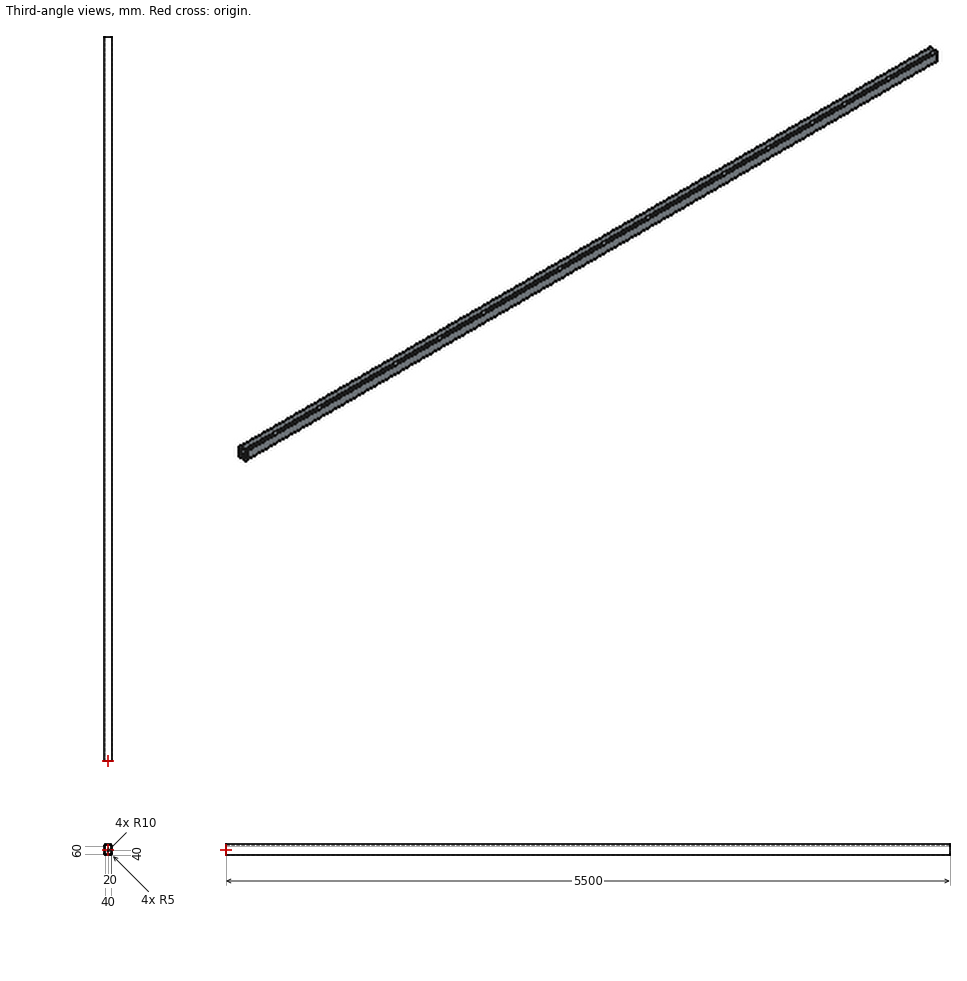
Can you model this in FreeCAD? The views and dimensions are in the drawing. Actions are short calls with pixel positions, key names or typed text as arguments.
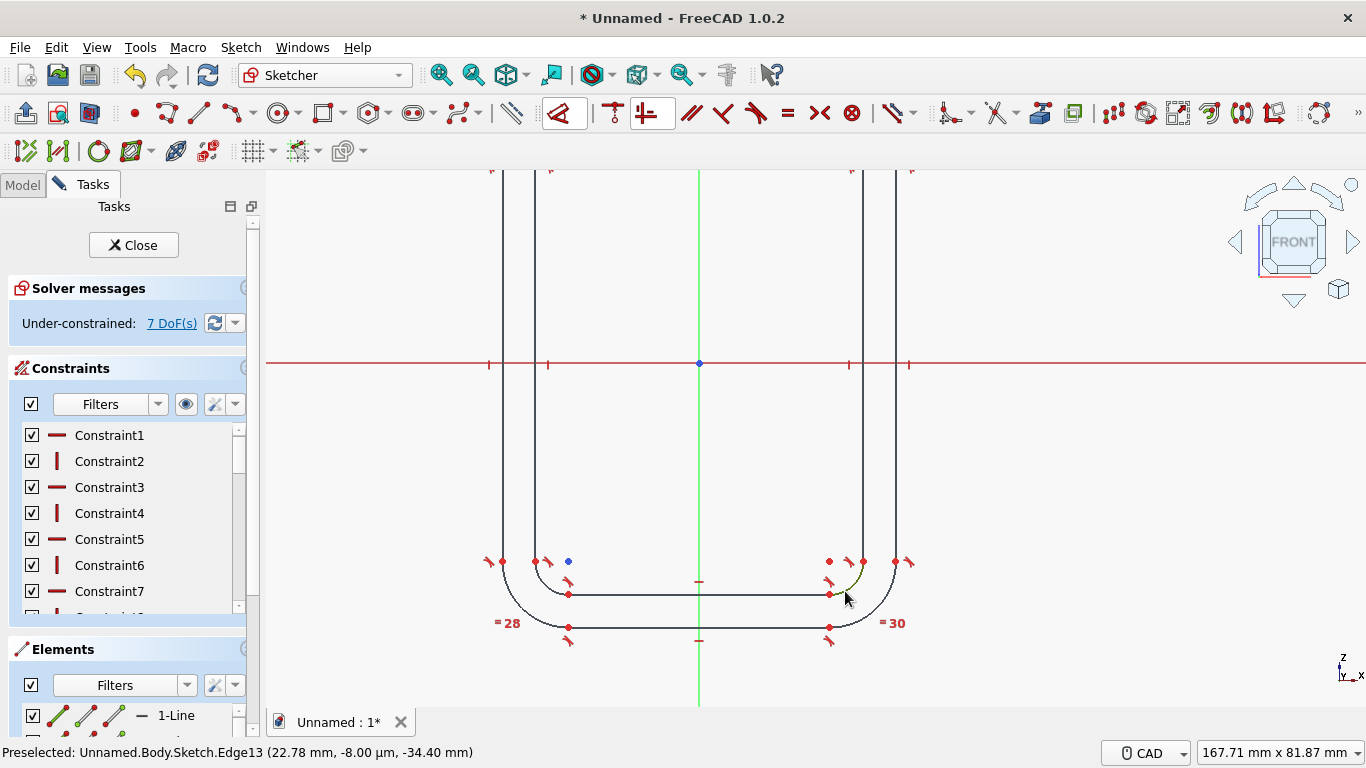
click(539, 577)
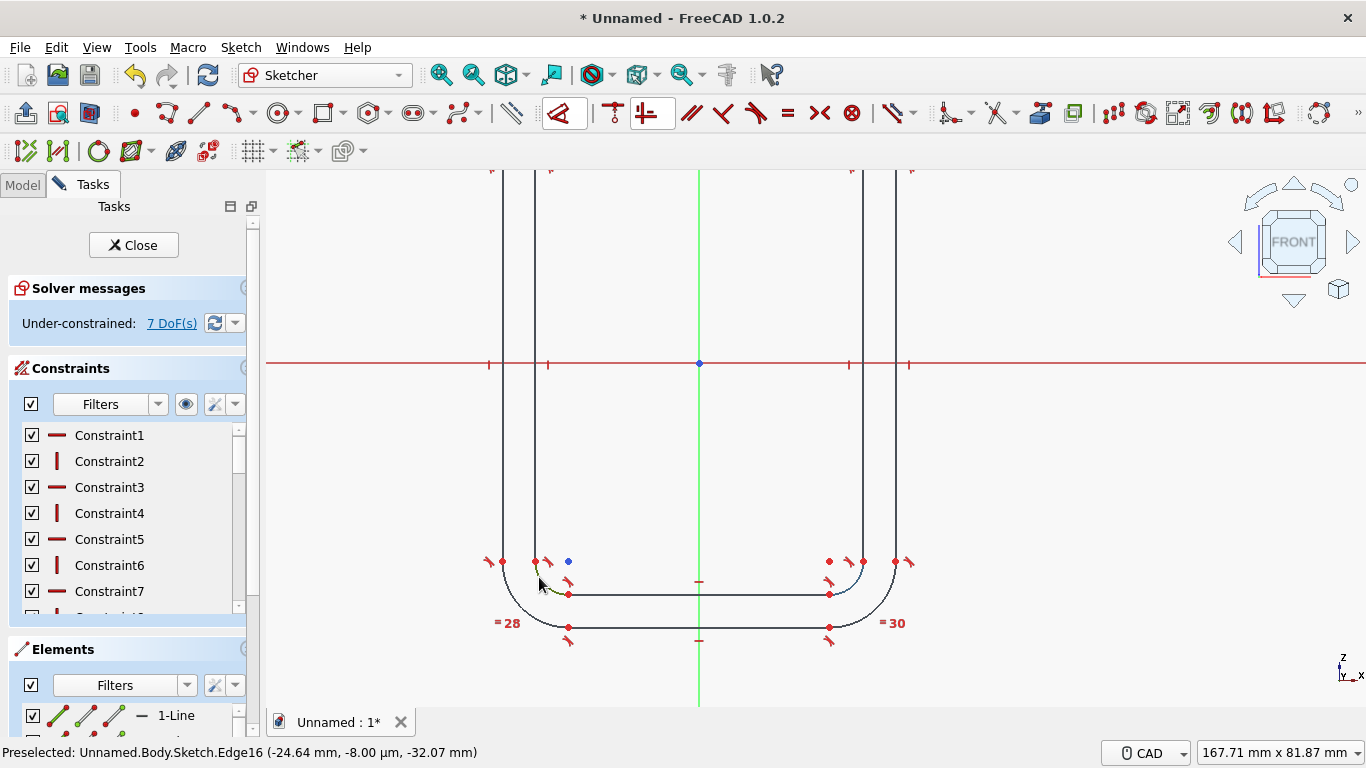
click(788, 114)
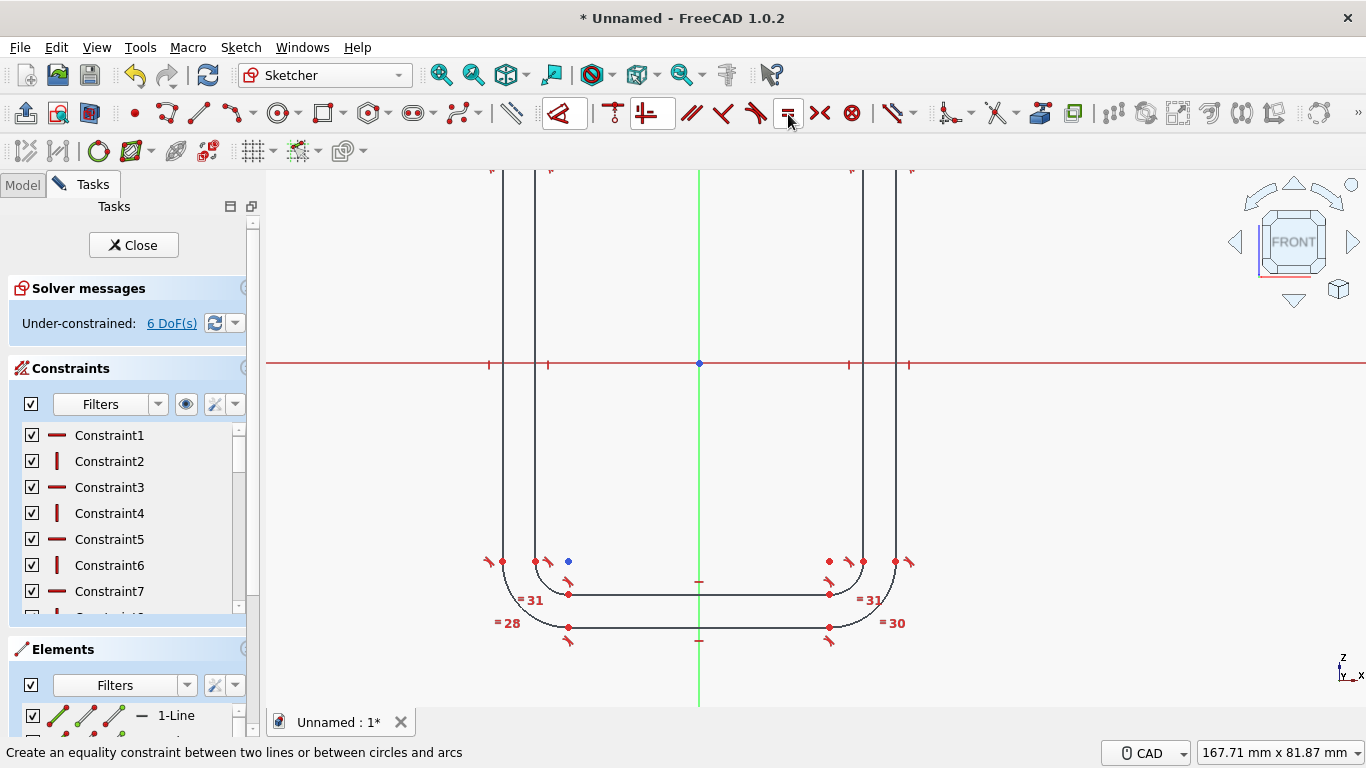
click(558, 114)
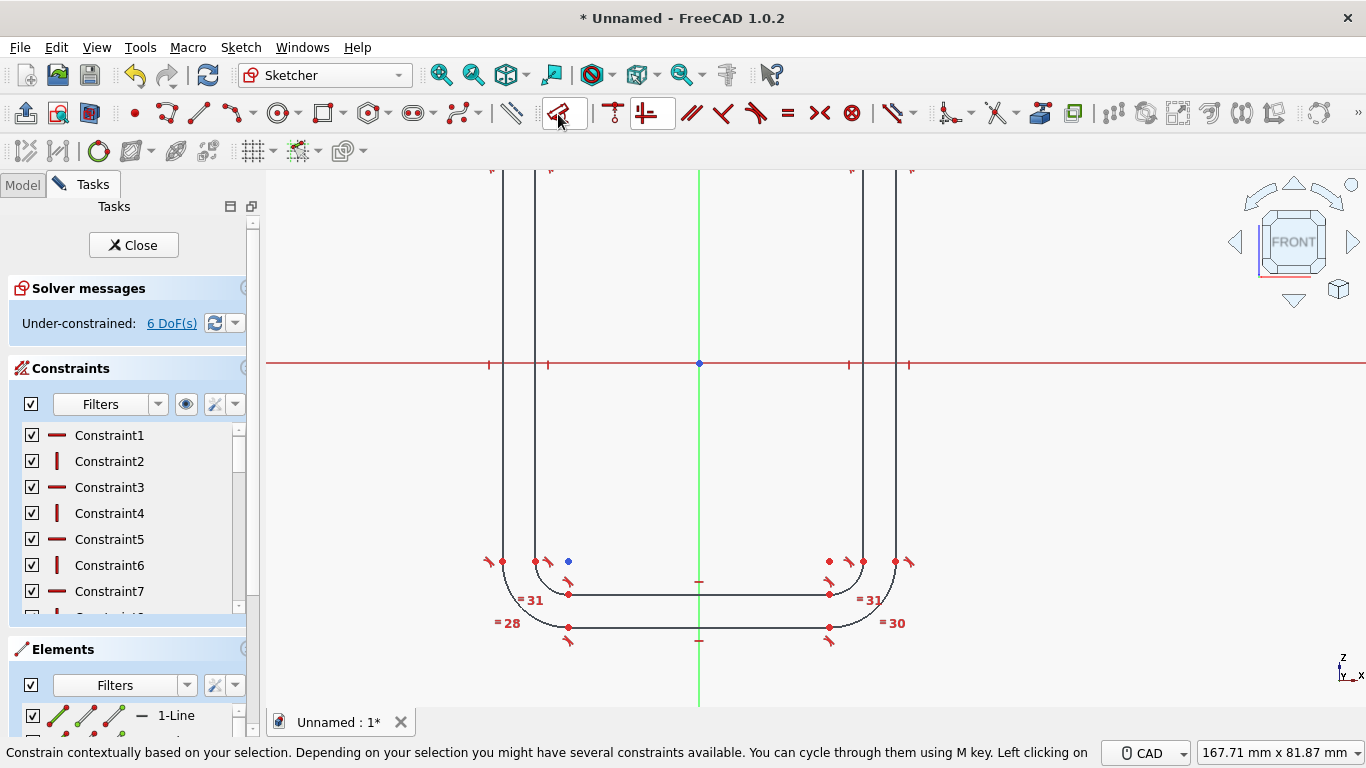
click(510, 592)
click(482, 607)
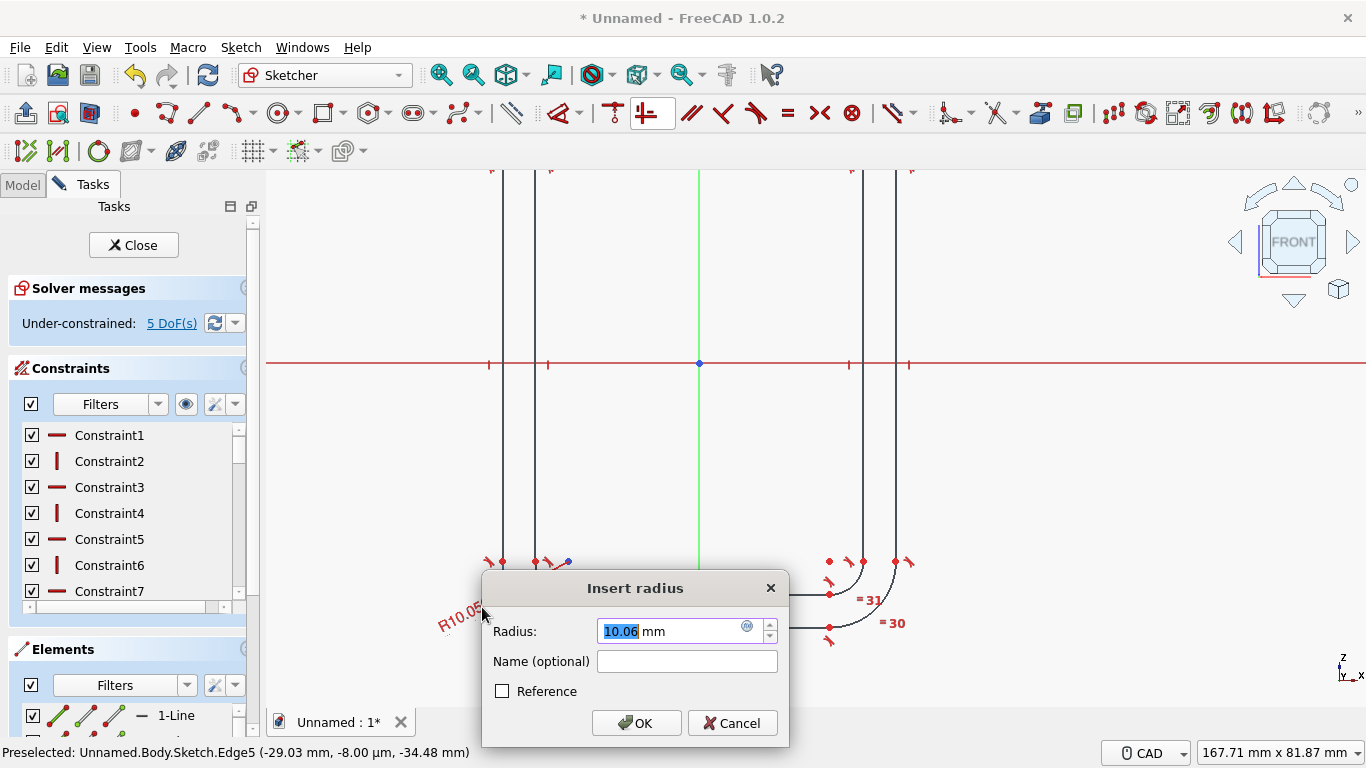
text(10)
key(Return)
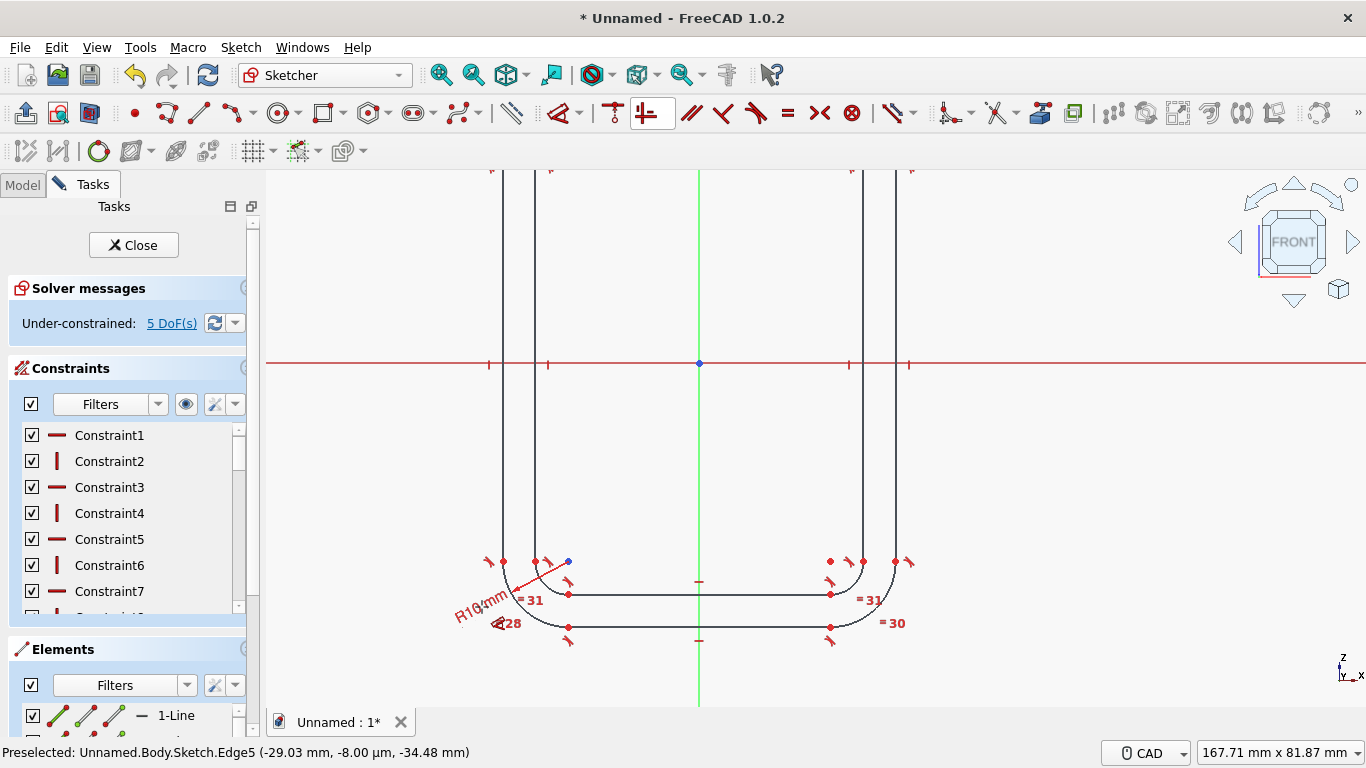
click(845, 591)
click(801, 504)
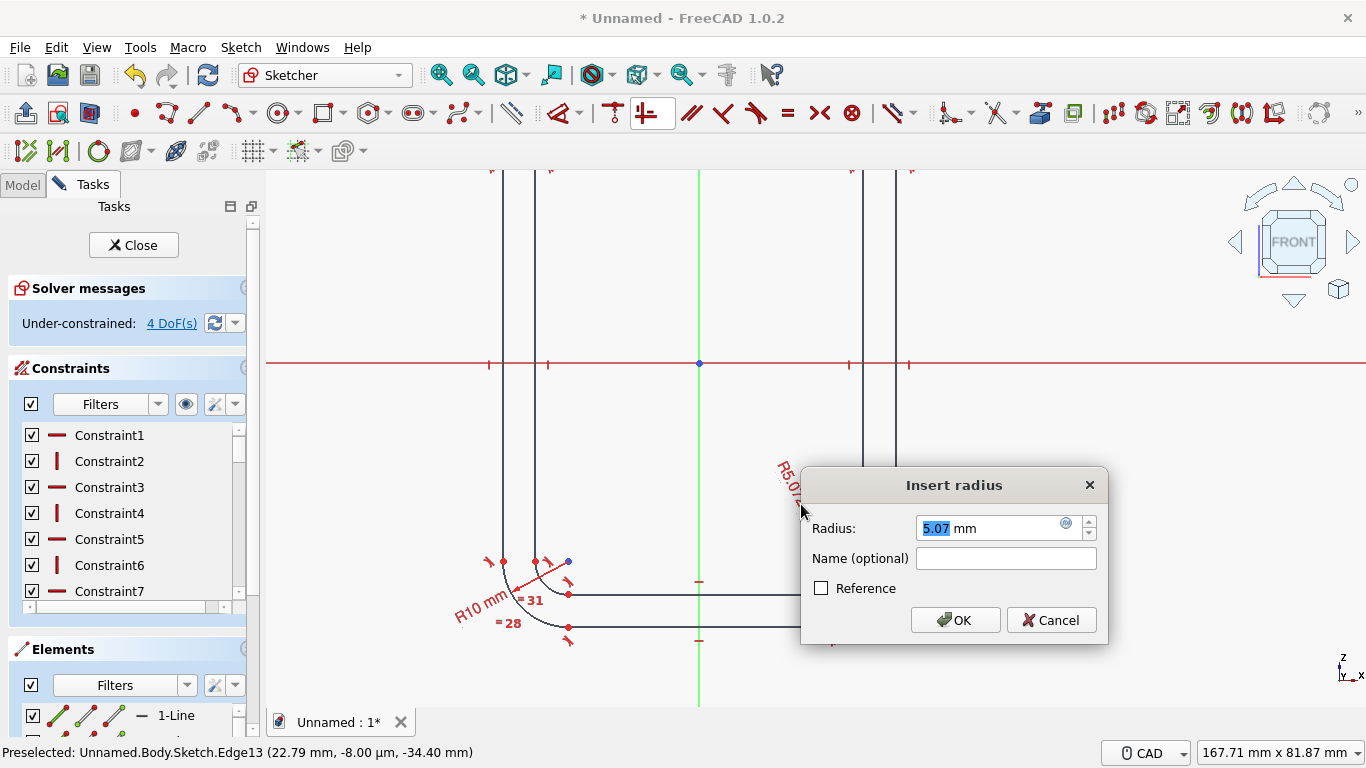
text(5)
key(Return)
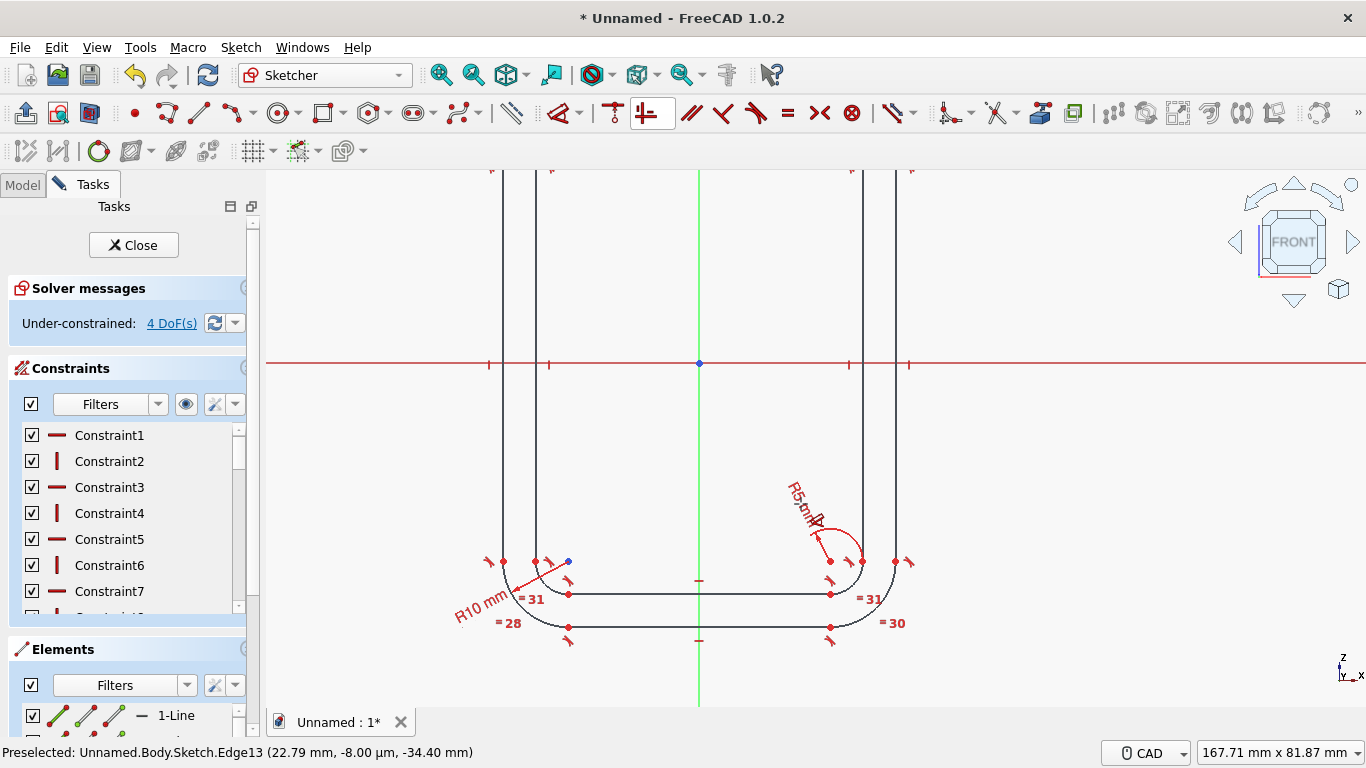
click(752, 627)
click(639, 661)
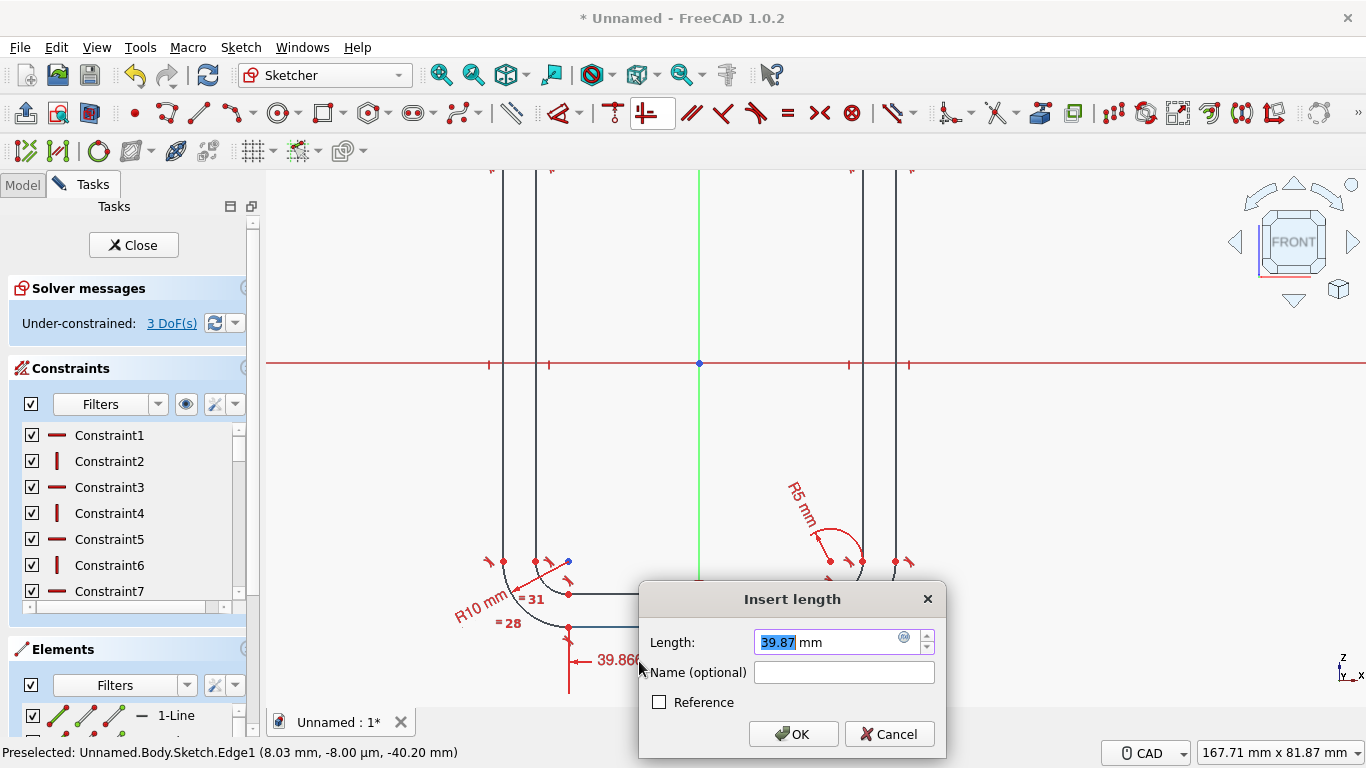
text(40)
key(Return)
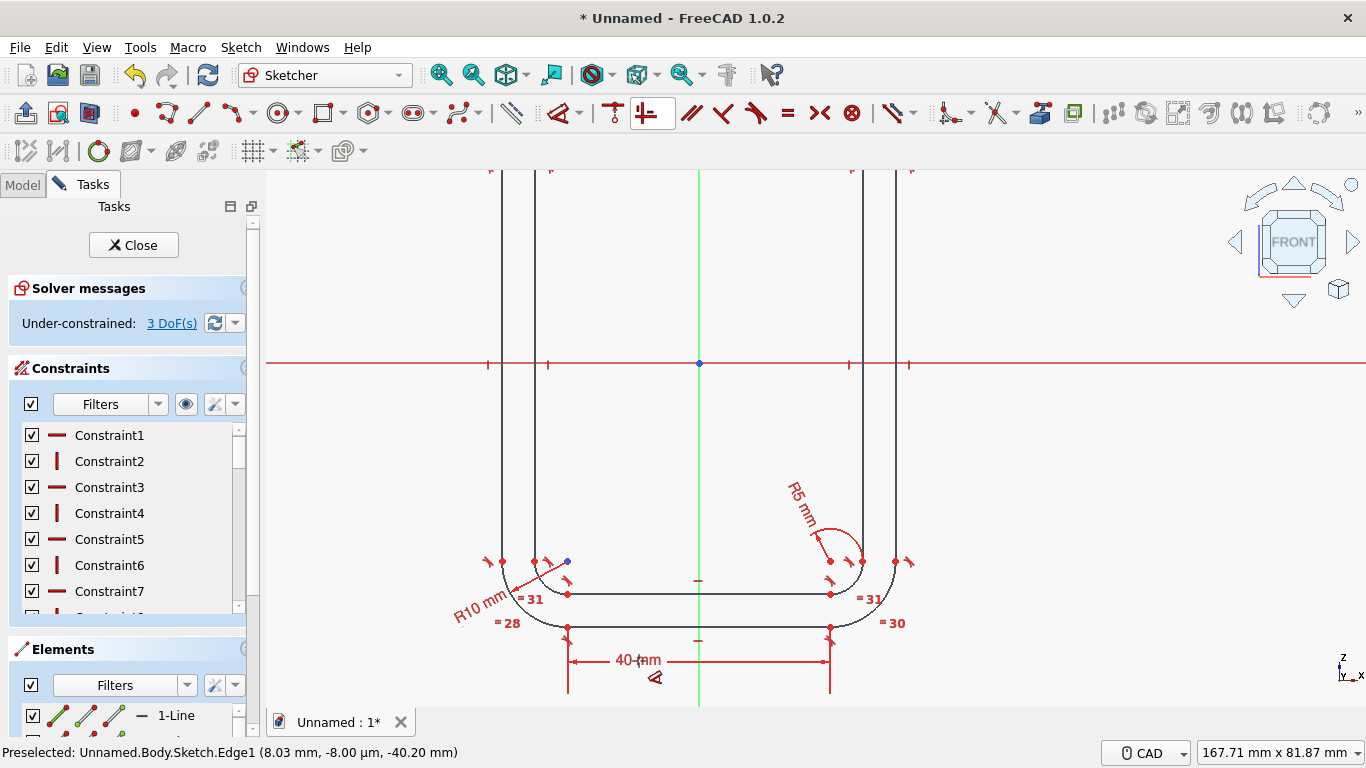
click(502, 443)
click(468, 380)